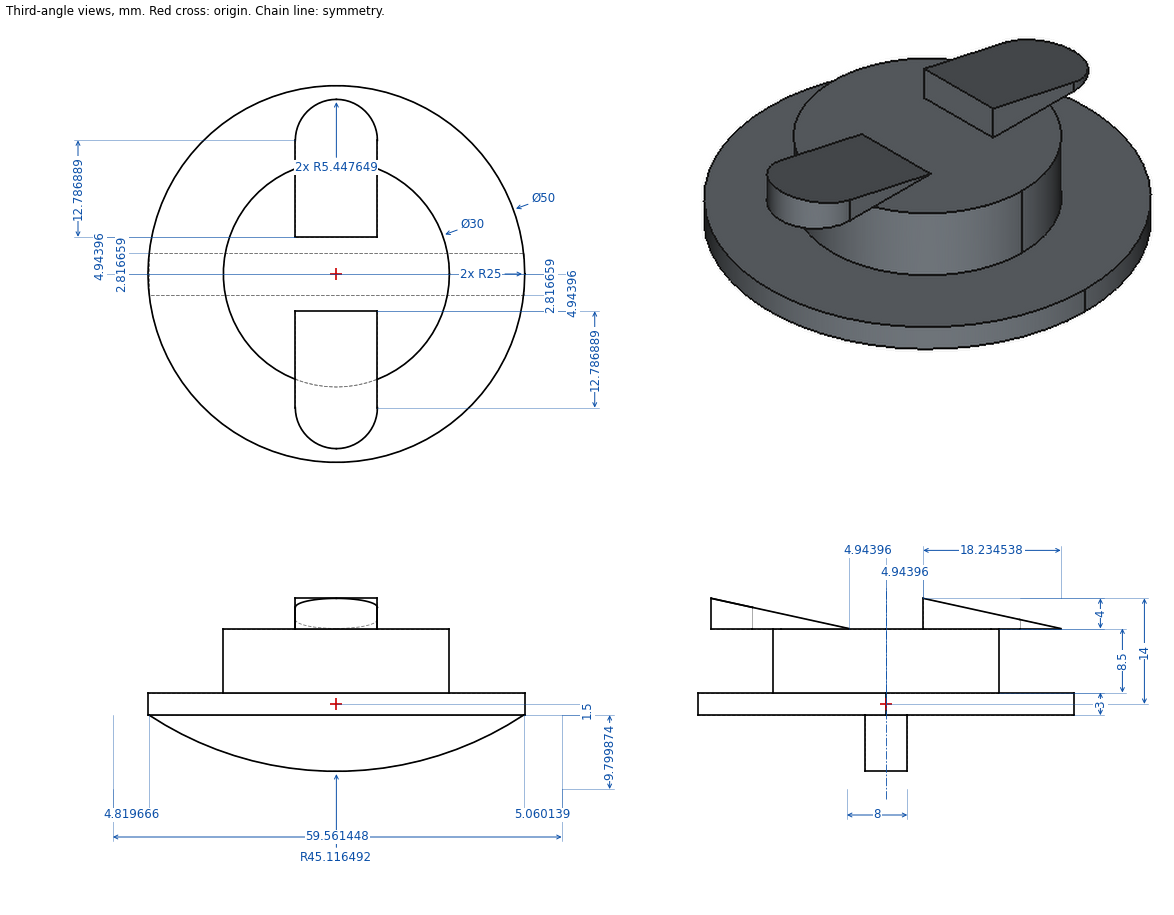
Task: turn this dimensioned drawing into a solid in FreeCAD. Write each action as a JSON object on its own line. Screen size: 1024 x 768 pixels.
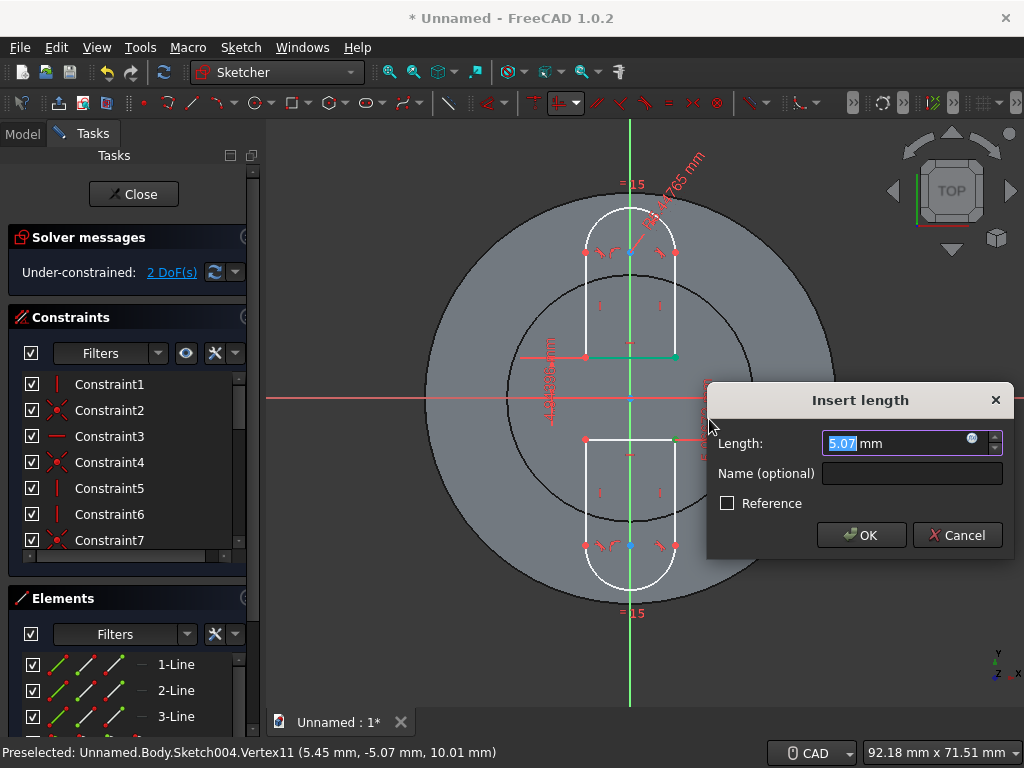
{"action": "type", "text": "4.94396"}
{"action": "key", "text": "Return"}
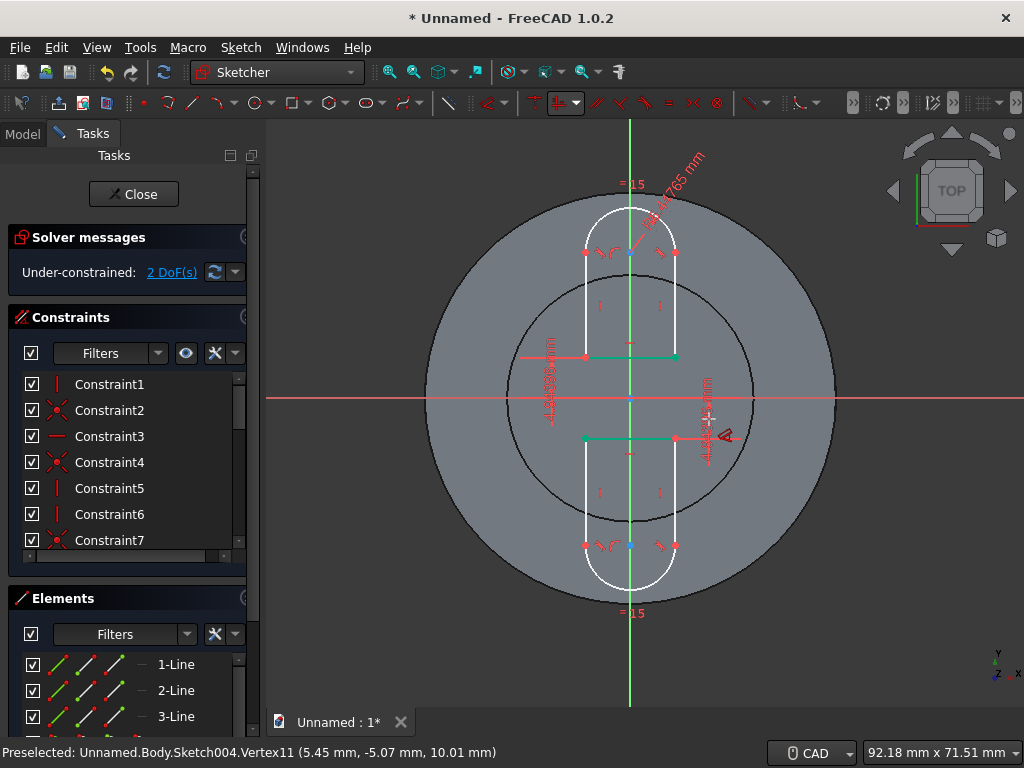
{"action": "left_click", "coordinate": [586, 284]}
{"action": "left_click", "coordinate": [552, 305]}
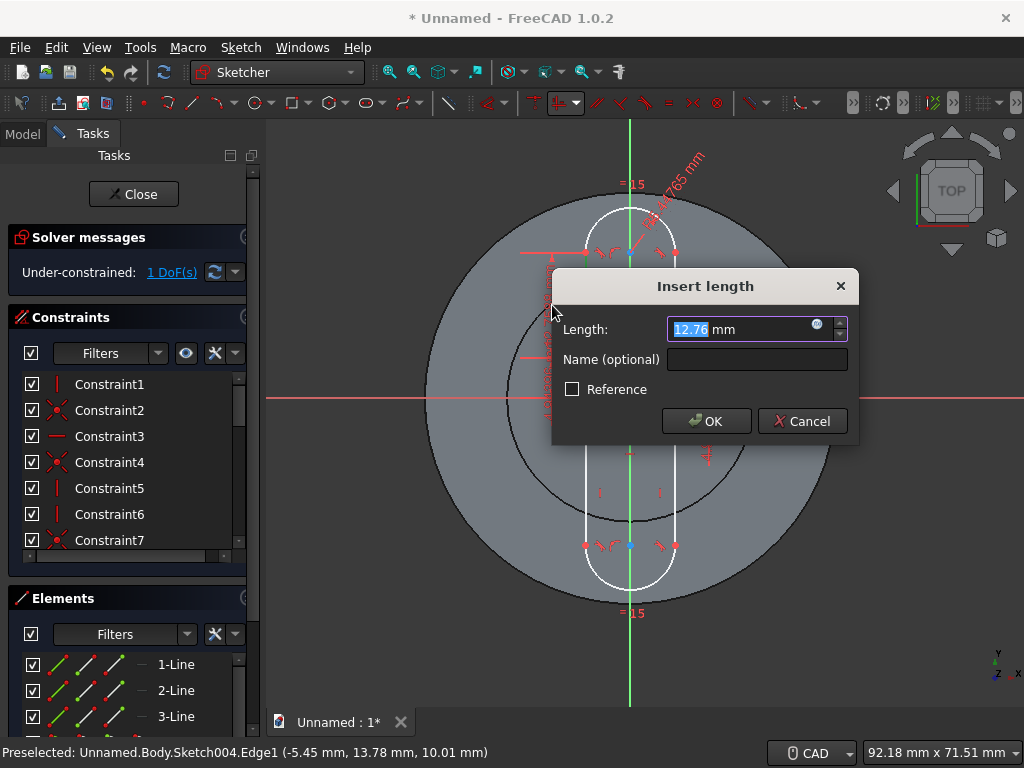
{"action": "type", "text": "12.786889"}
{"action": "key", "text": "Return"}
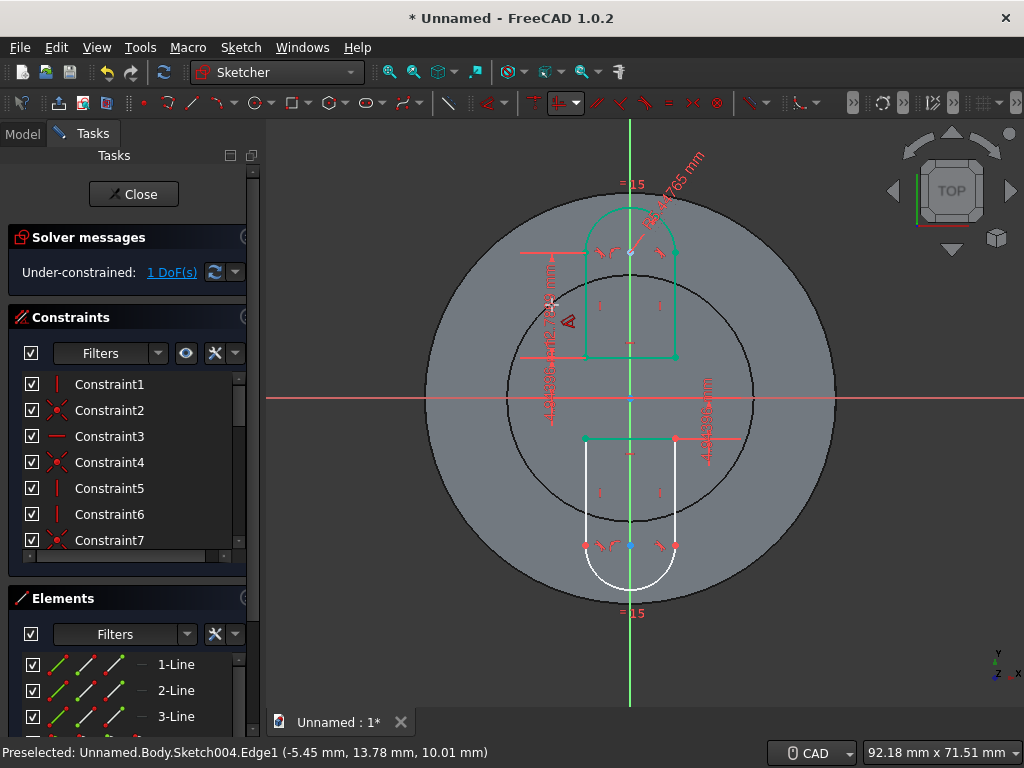
{"action": "left_click", "coordinate": [675, 513]}
{"action": "left_click", "coordinate": [709, 492]}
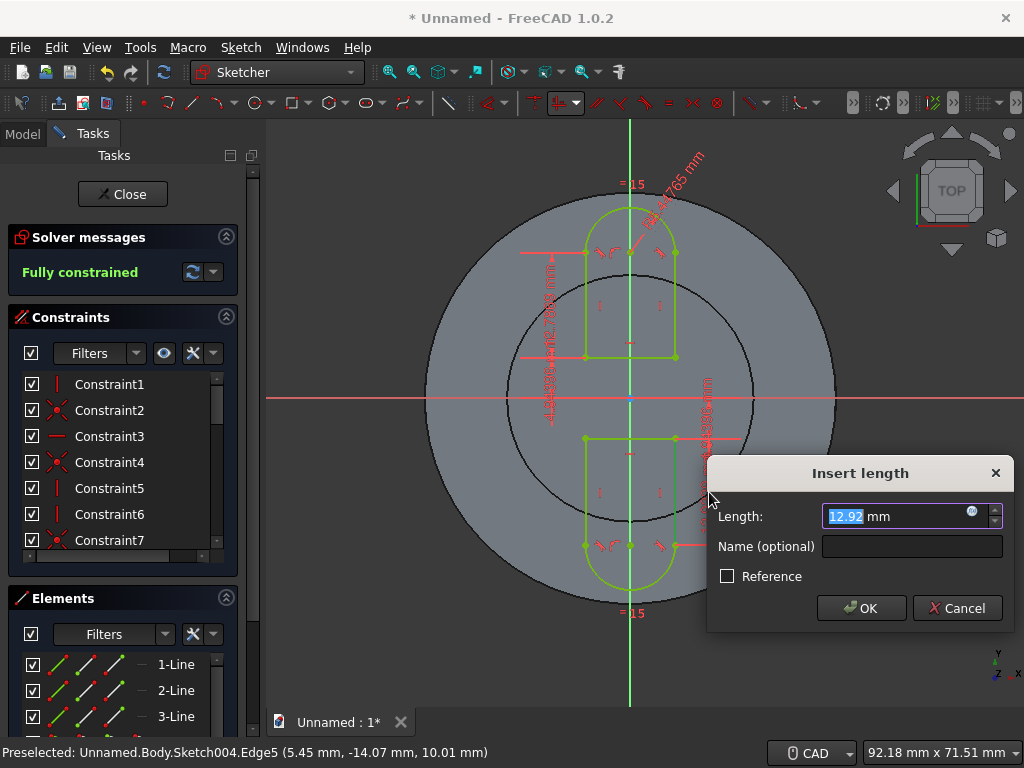
{"action": "type", "text": "12.786889"}
{"action": "key", "text": "Return"}
{"action": "key", "text": "Escape"}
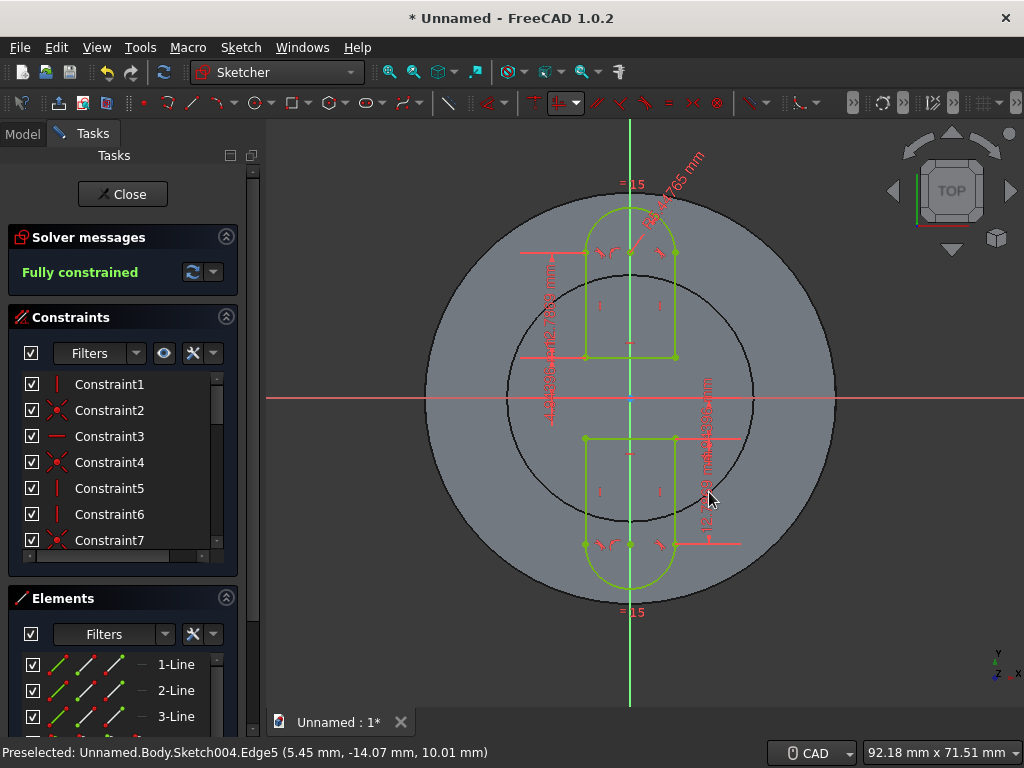
{"action": "left_click", "coordinate": [123, 194]}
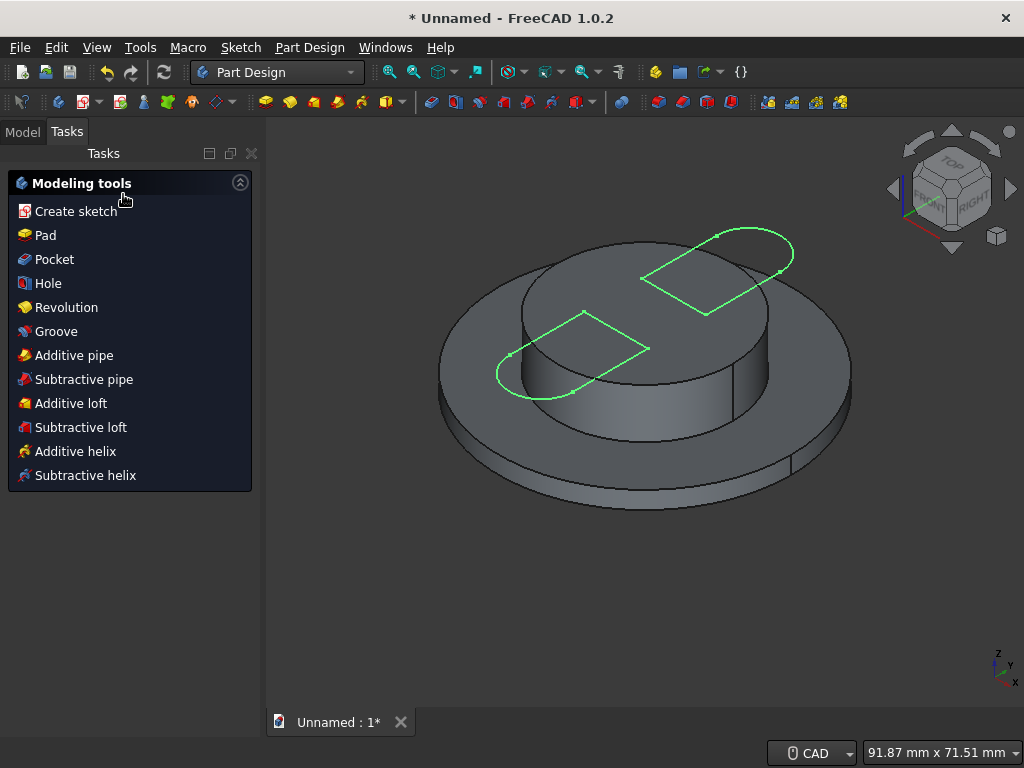
{"action": "left_click", "coordinate": [266, 102]}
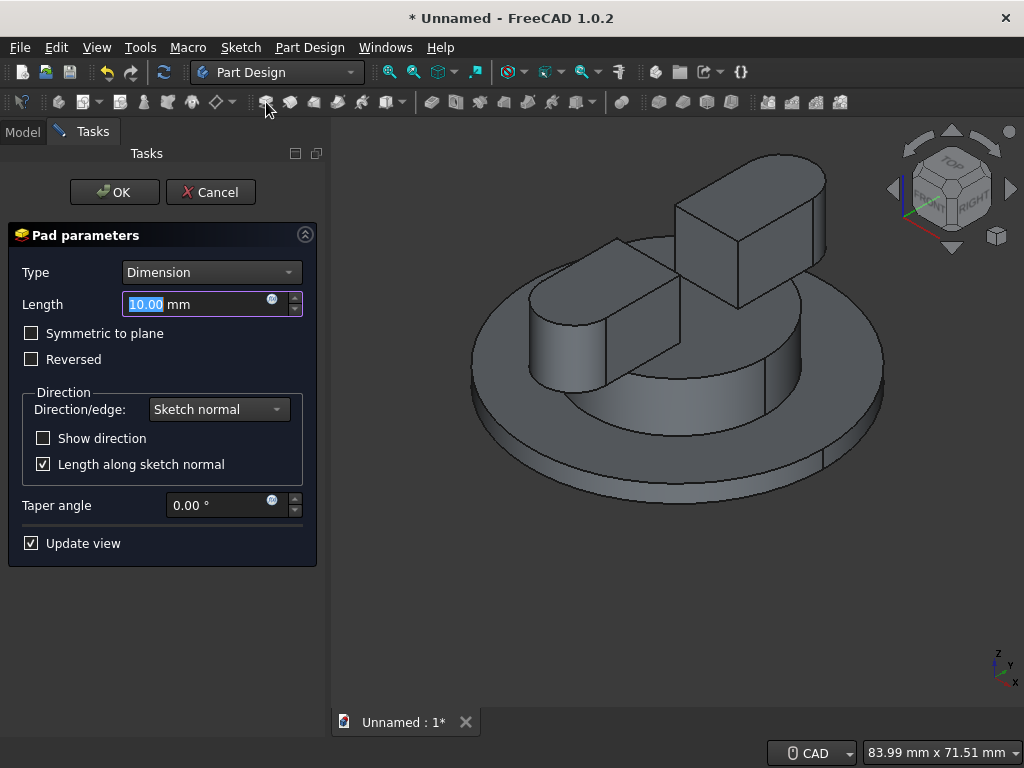
{"action": "type", "text": "4"}
{"action": "key", "text": "Tab"}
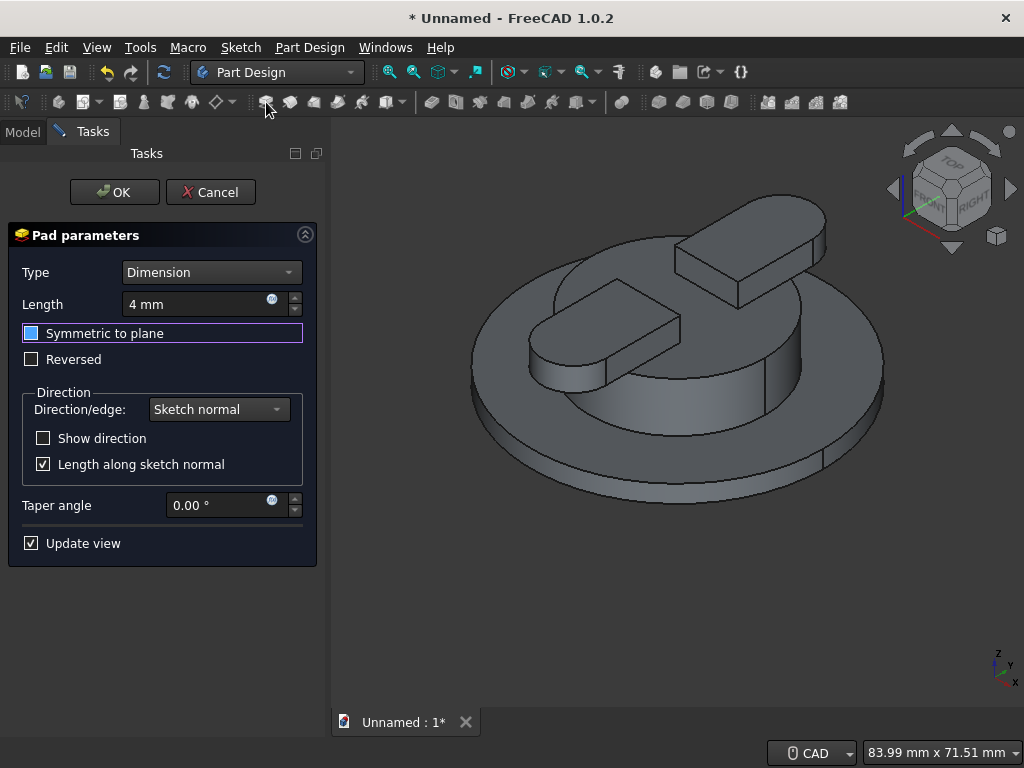
{"action": "left_click", "coordinate": [115, 192]}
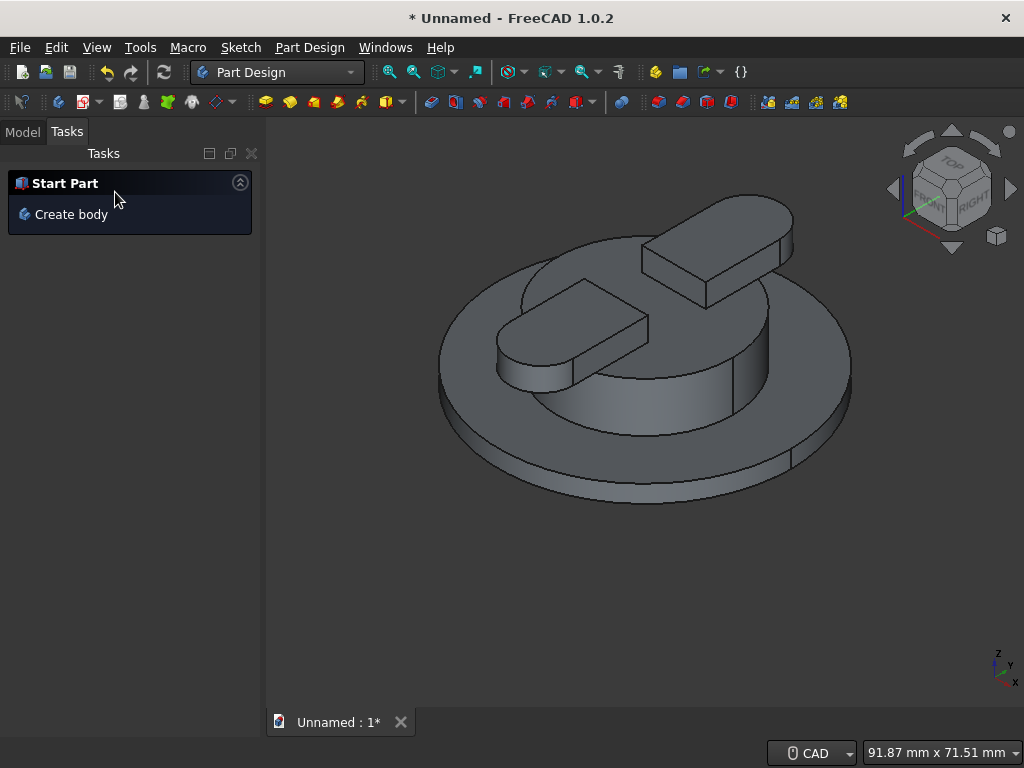
{"action": "left_click", "coordinate": [390, 72]}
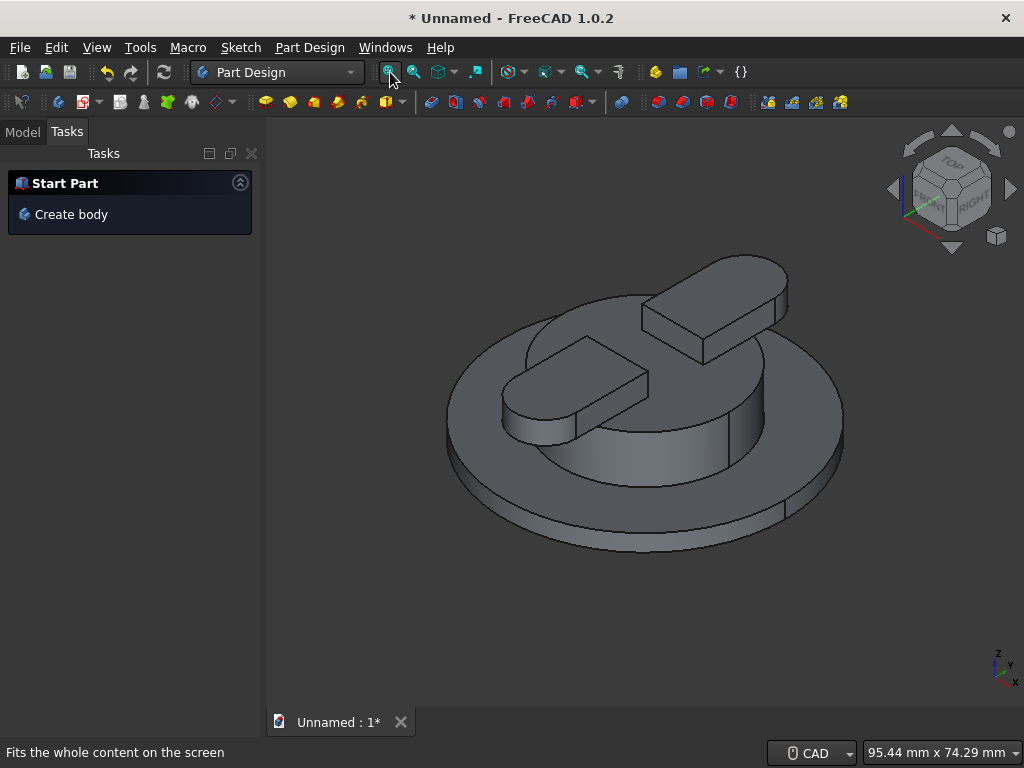
{"action": "key", "text": "6"}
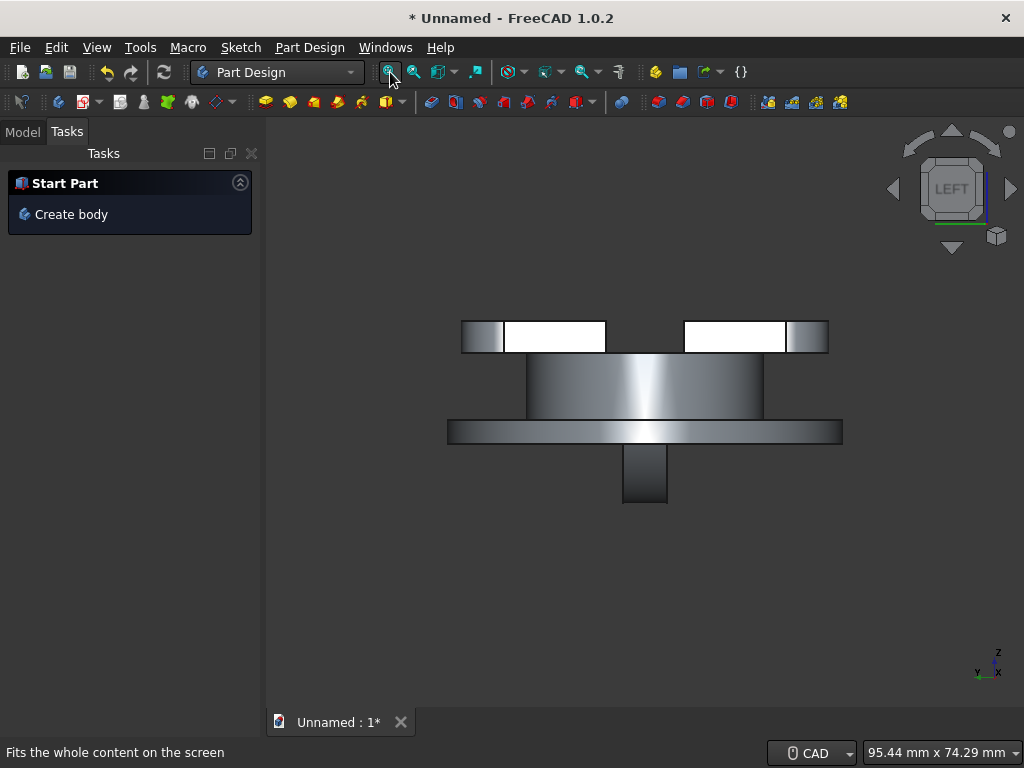
{"action": "left_click", "coordinate": [706, 336]}